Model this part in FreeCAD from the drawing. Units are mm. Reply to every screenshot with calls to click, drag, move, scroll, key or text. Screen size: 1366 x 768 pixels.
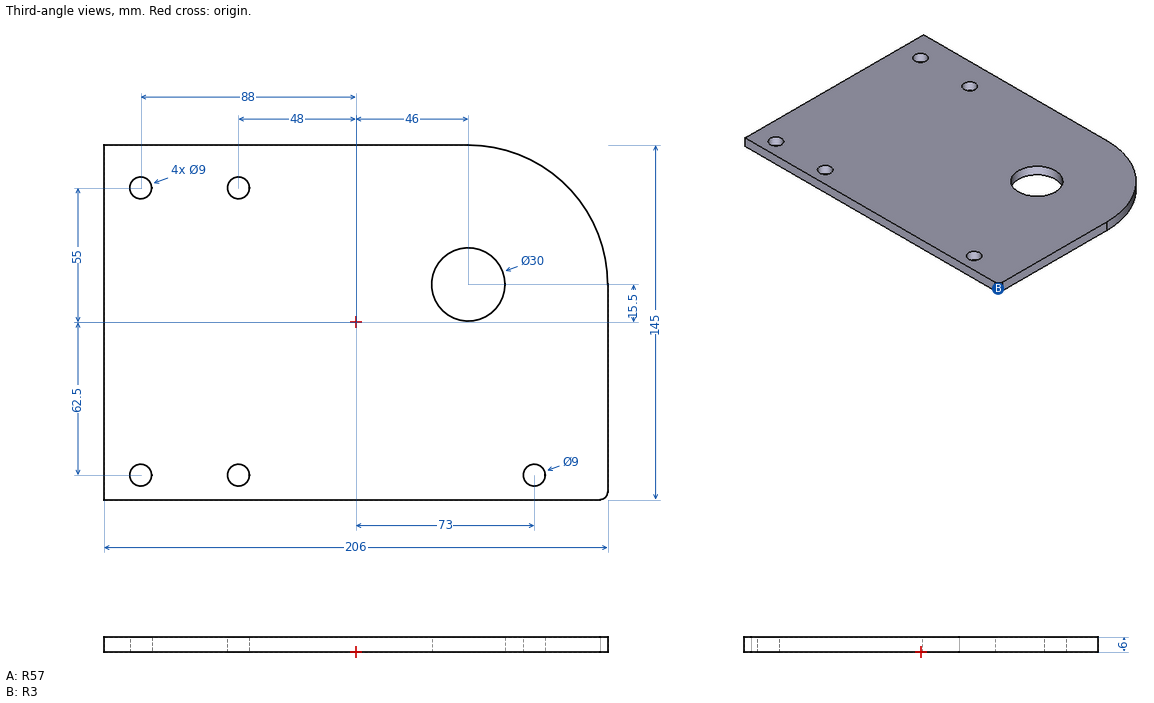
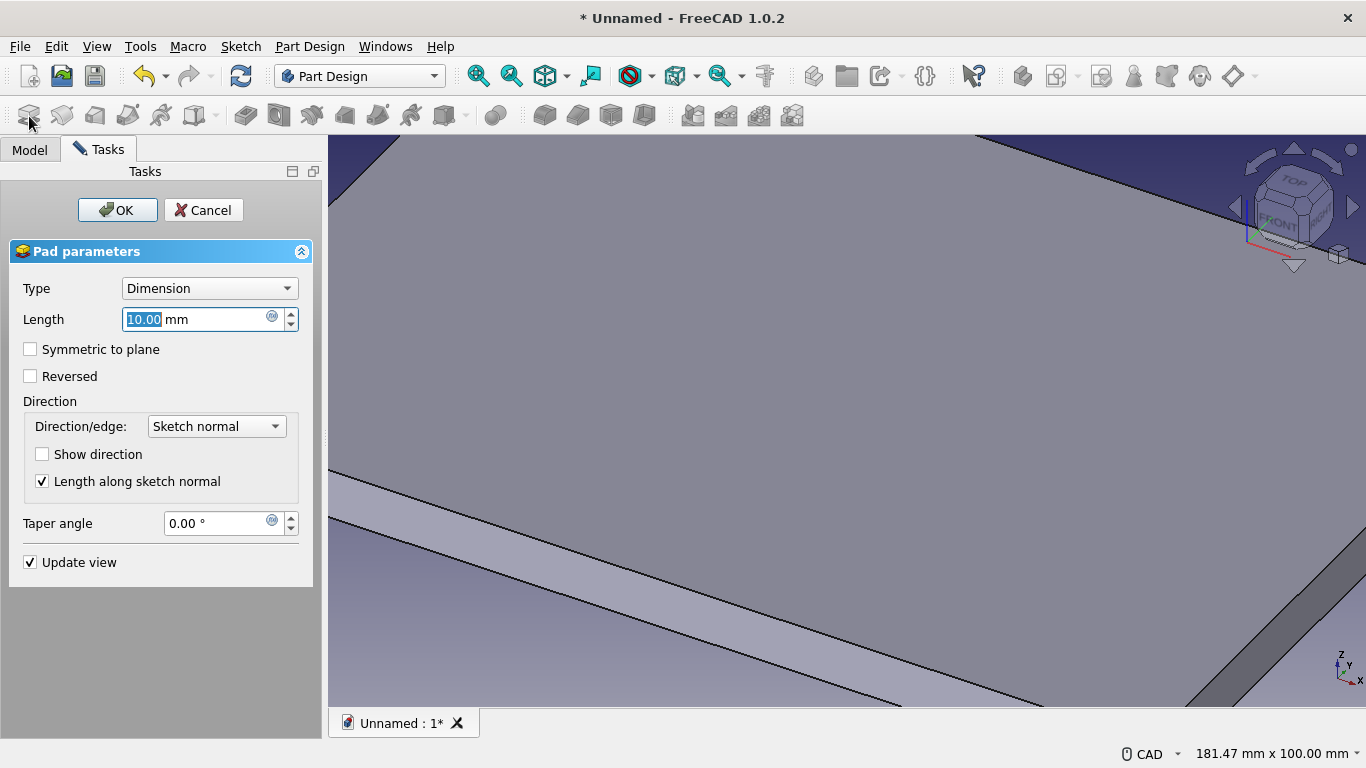
text(6)
key(Tab)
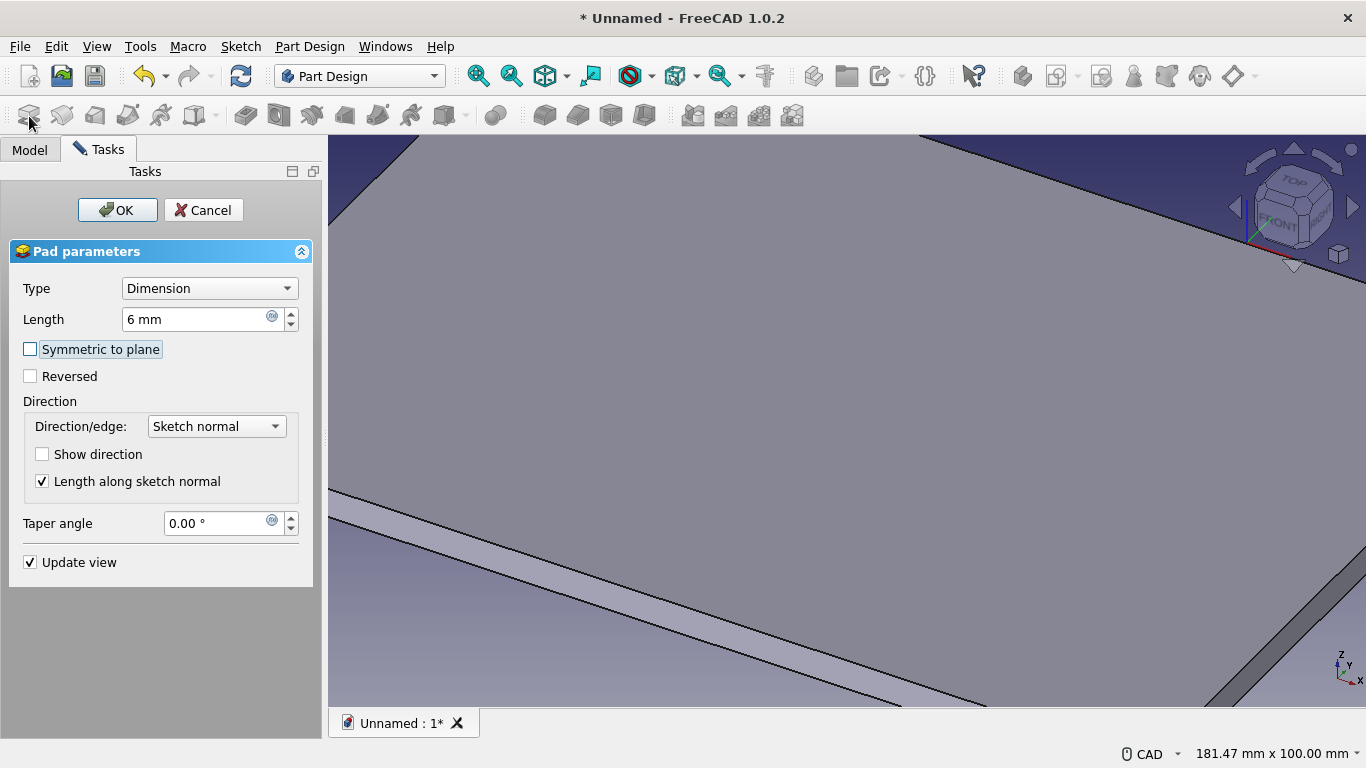
click(118, 210)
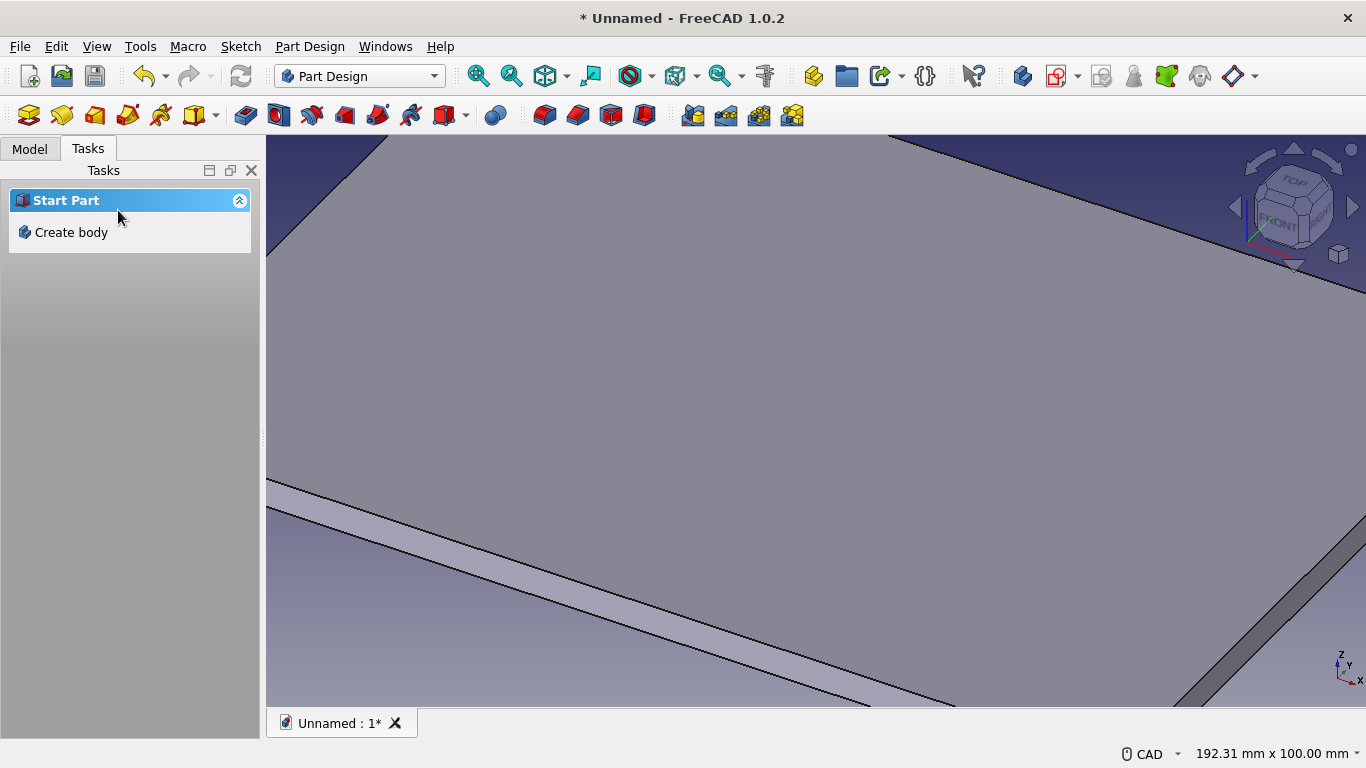
click(479, 76)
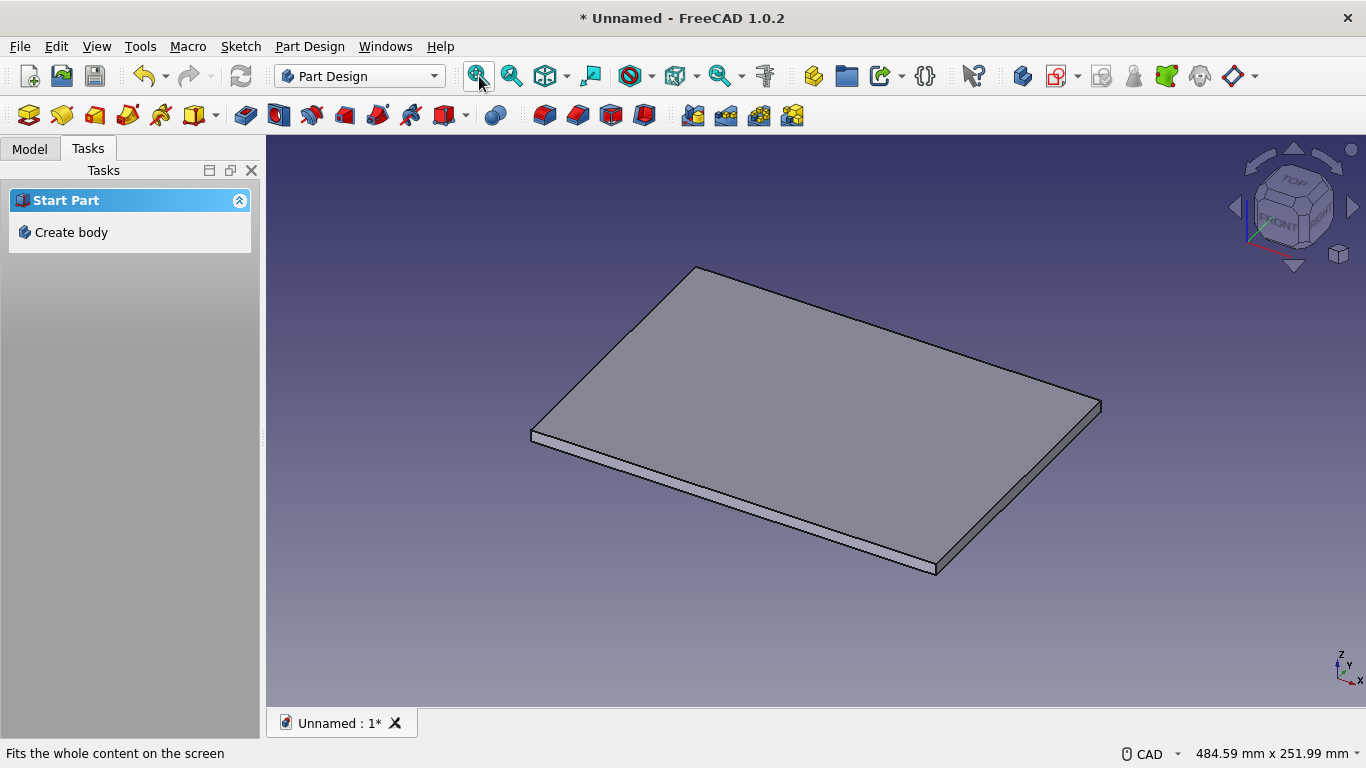
click(874, 434)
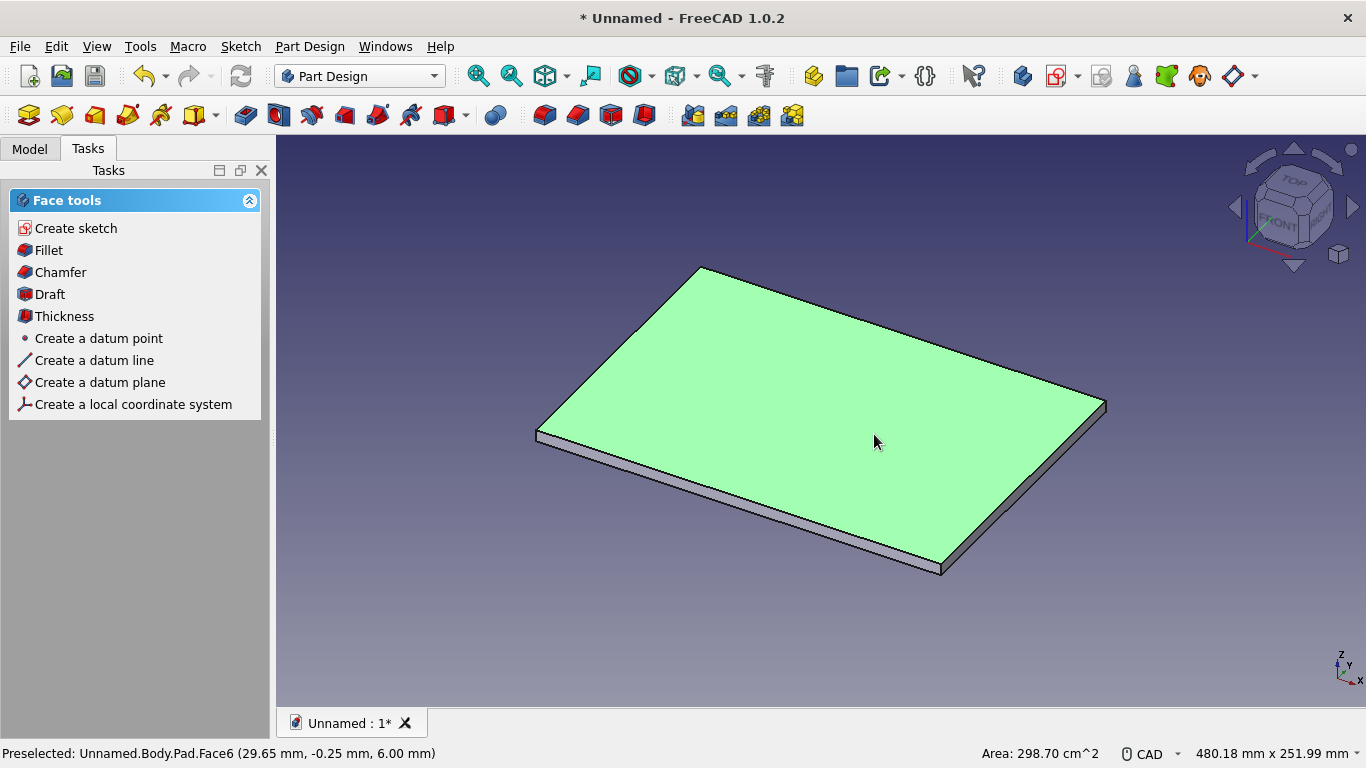
click(1056, 76)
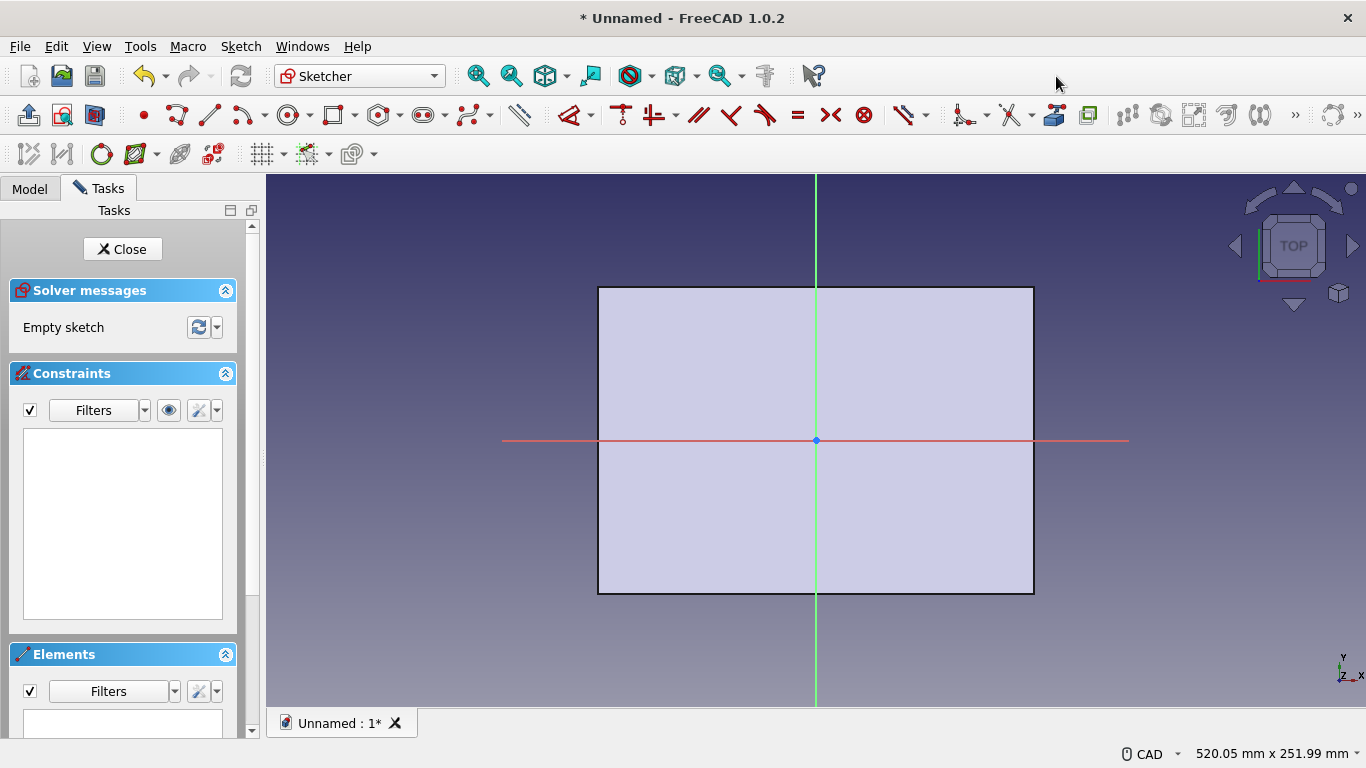
key(g)
key(c)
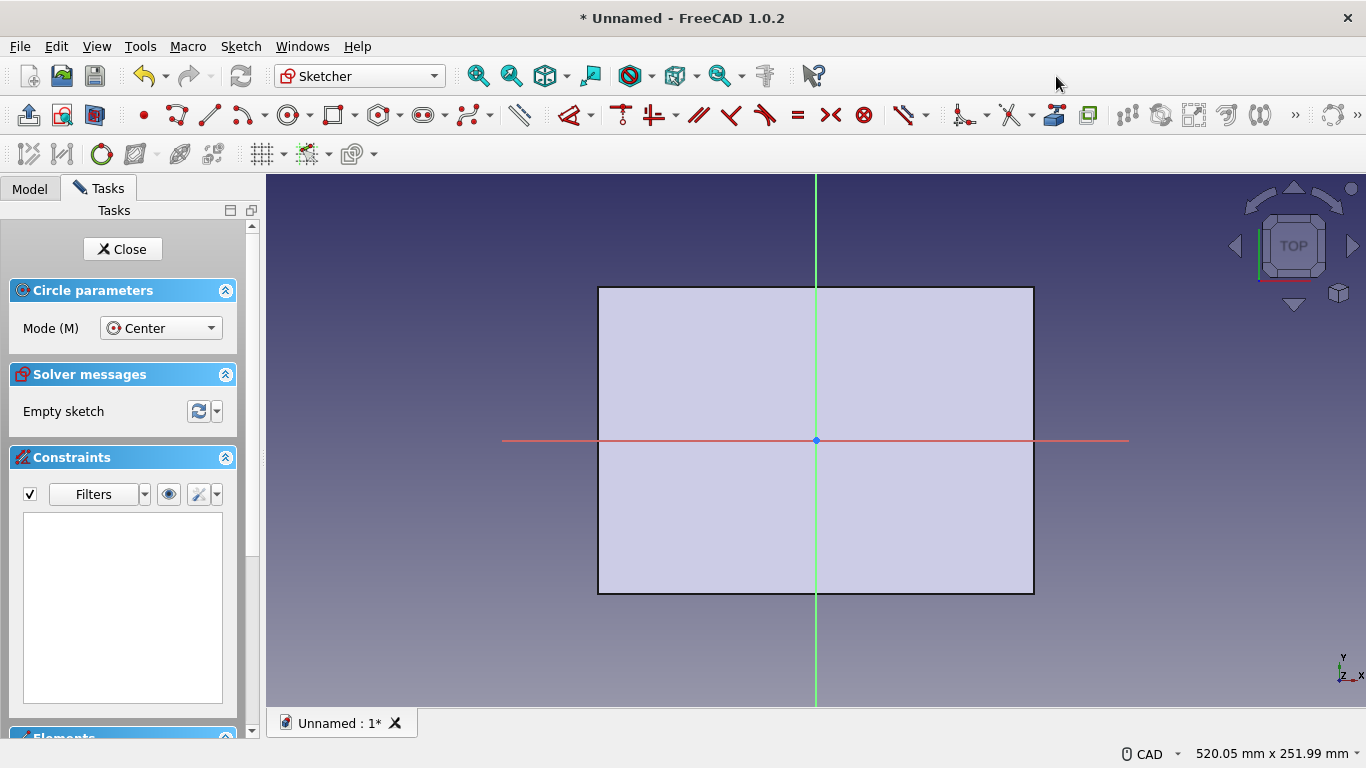
scroll(630, 324, up, 5)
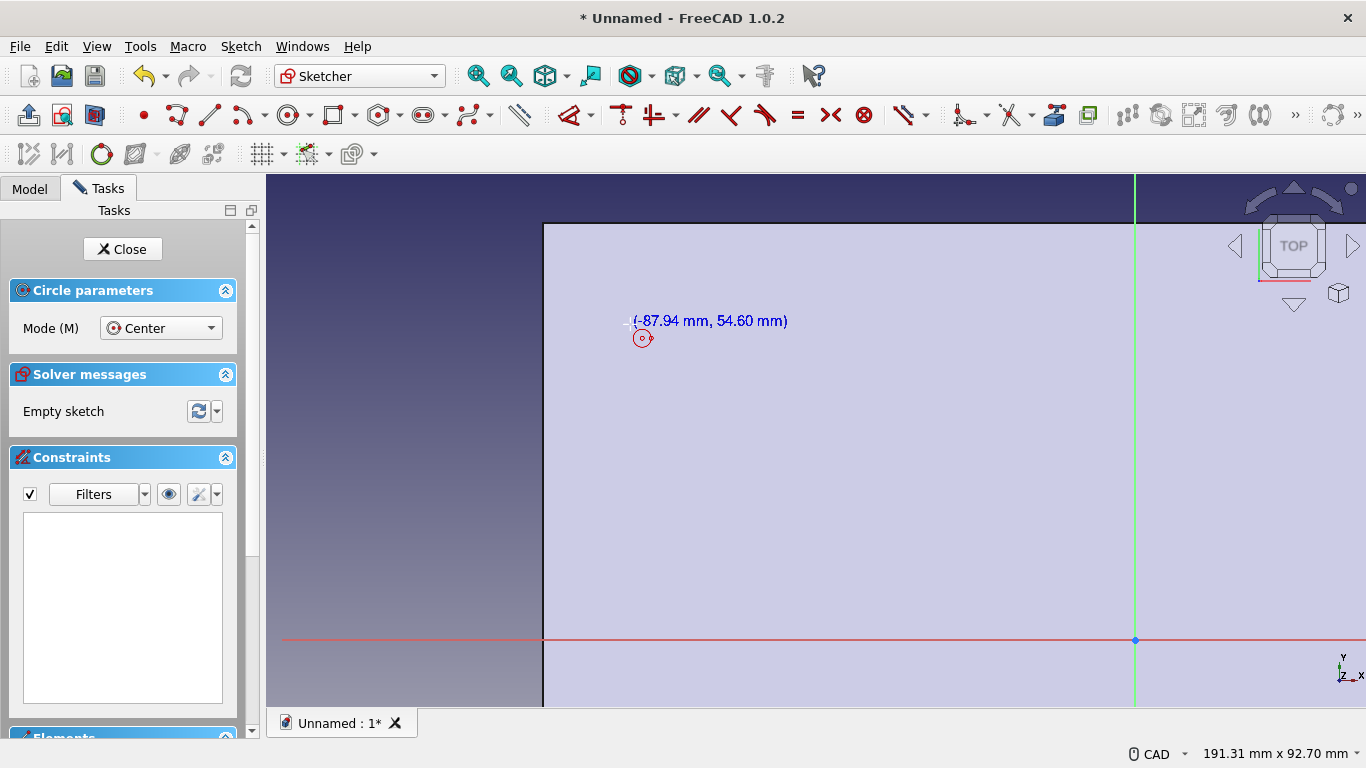
click(629, 324)
move(647, 306)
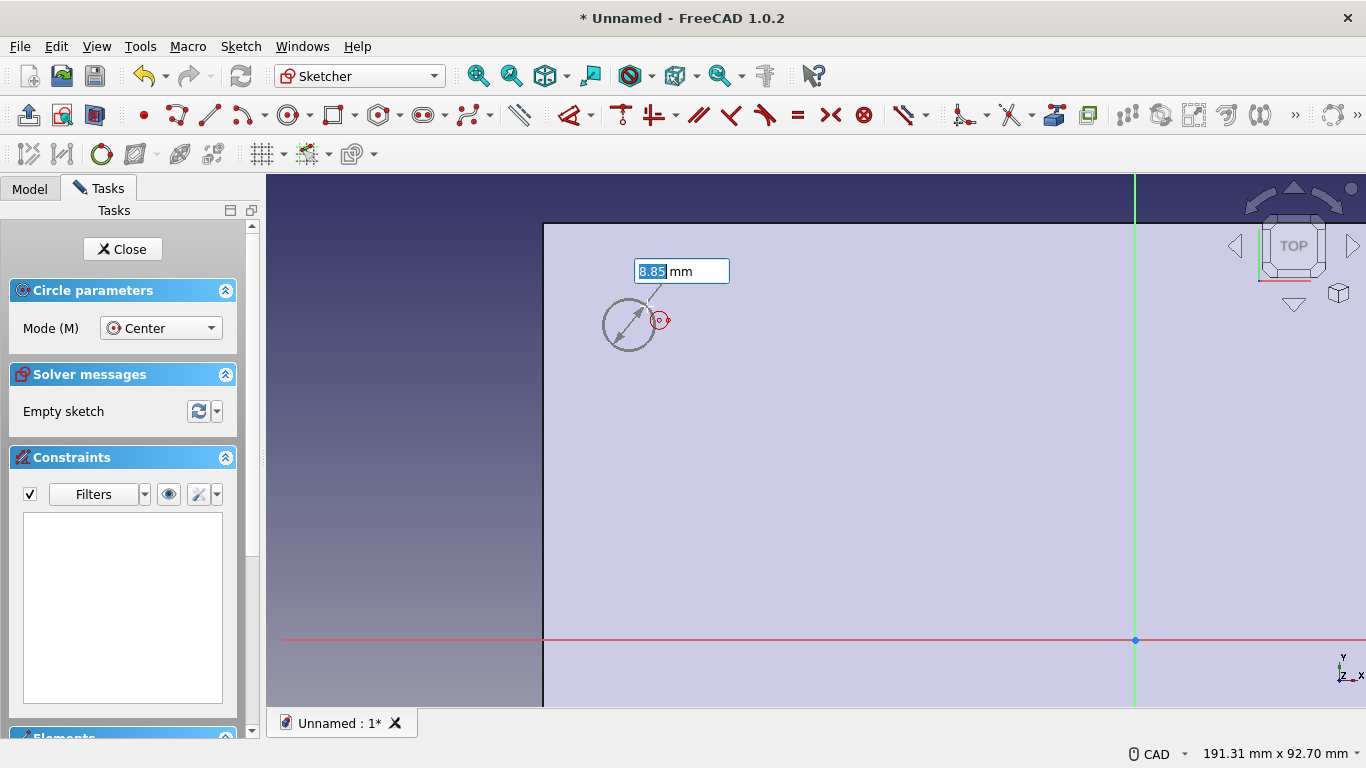
text(9)
key(Return)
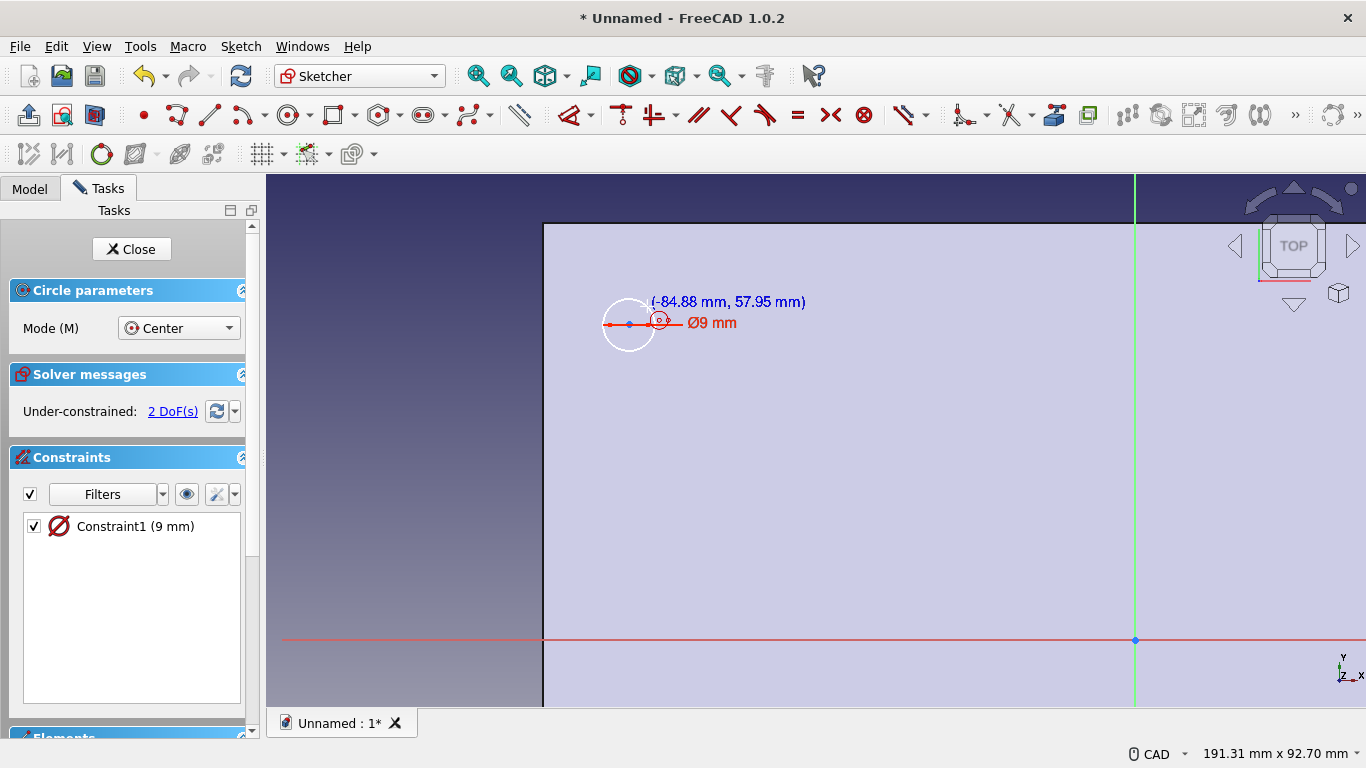
click(859, 324)
move(877, 306)